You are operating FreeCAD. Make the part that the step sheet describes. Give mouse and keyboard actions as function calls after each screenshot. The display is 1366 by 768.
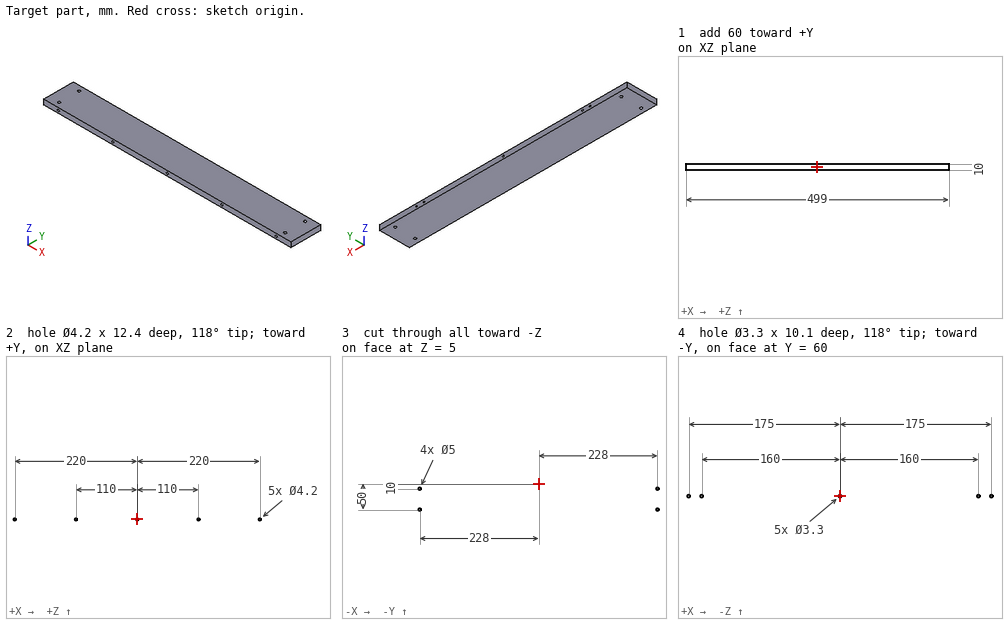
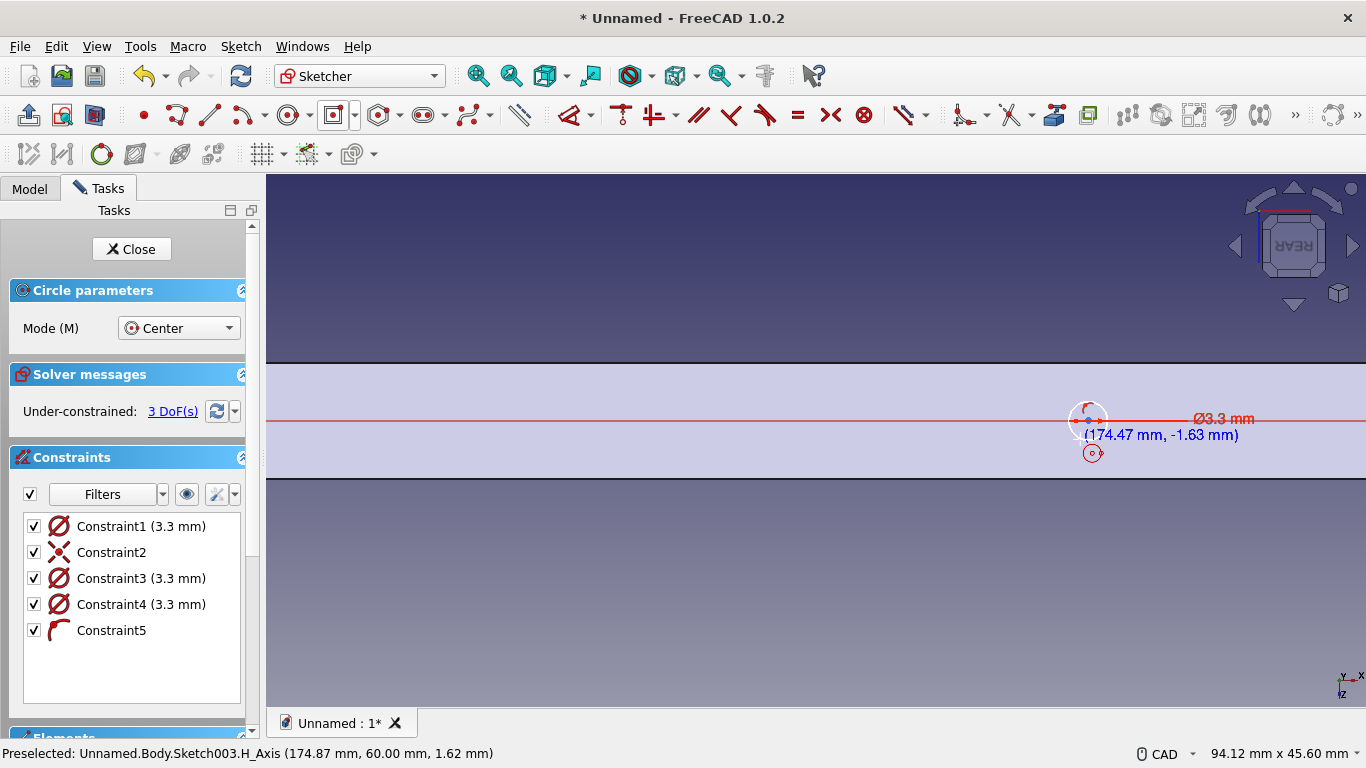
scroll(1085, 444, down, 9)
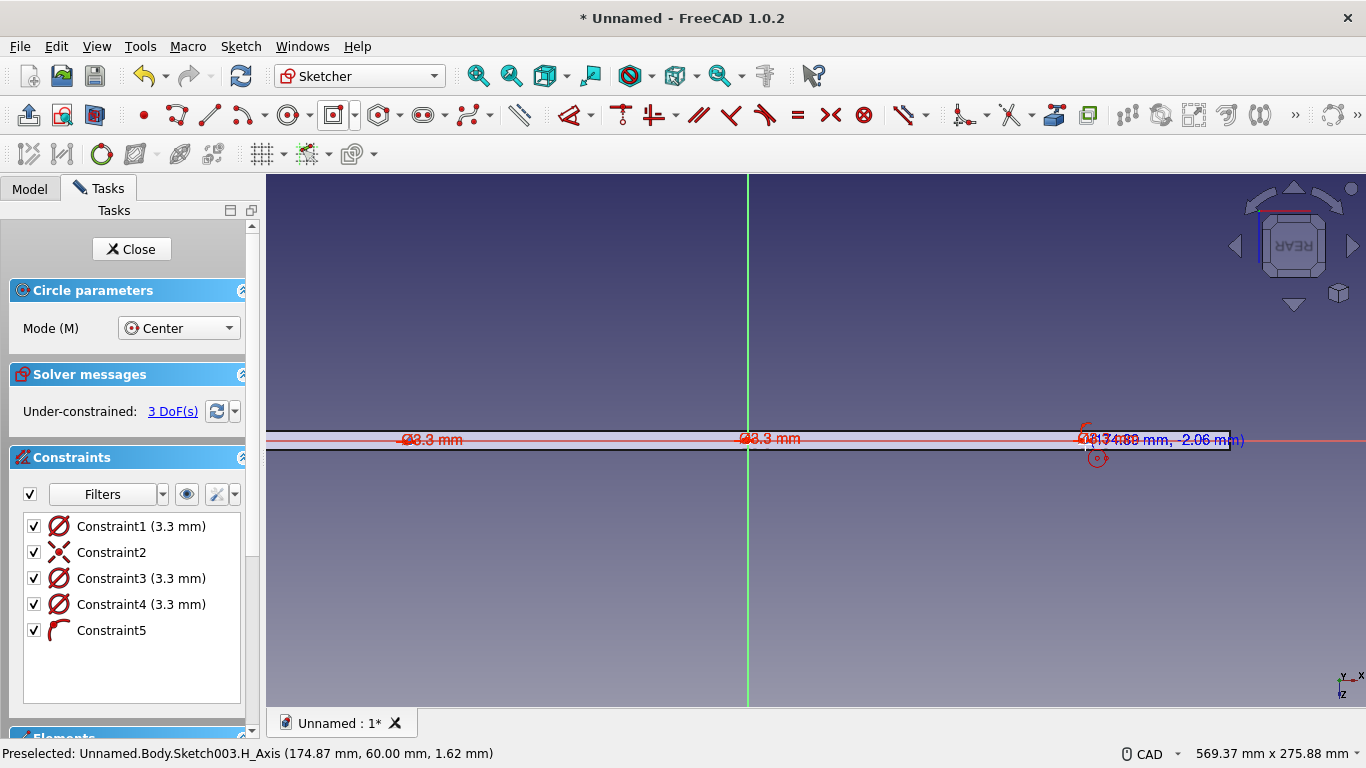
scroll(439, 441, up, 10)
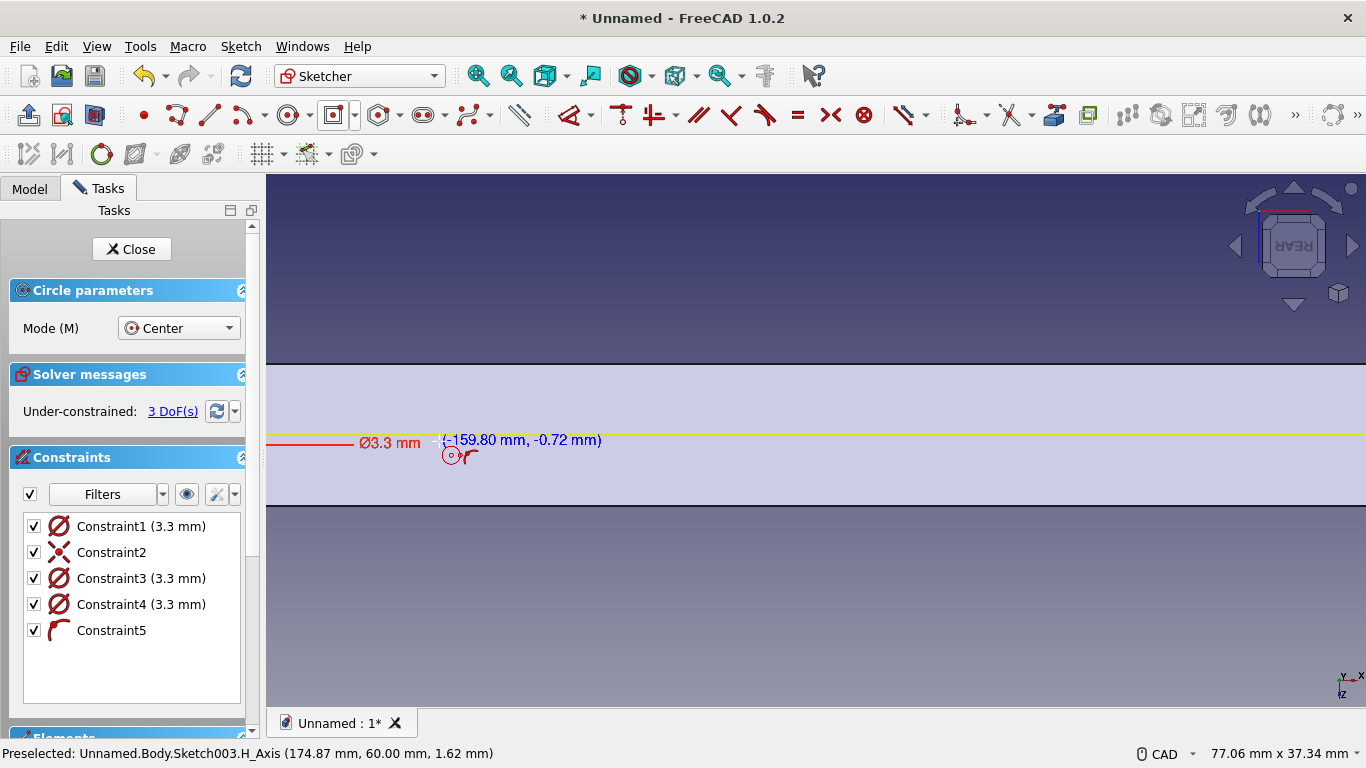
scroll(439, 441, down, 10)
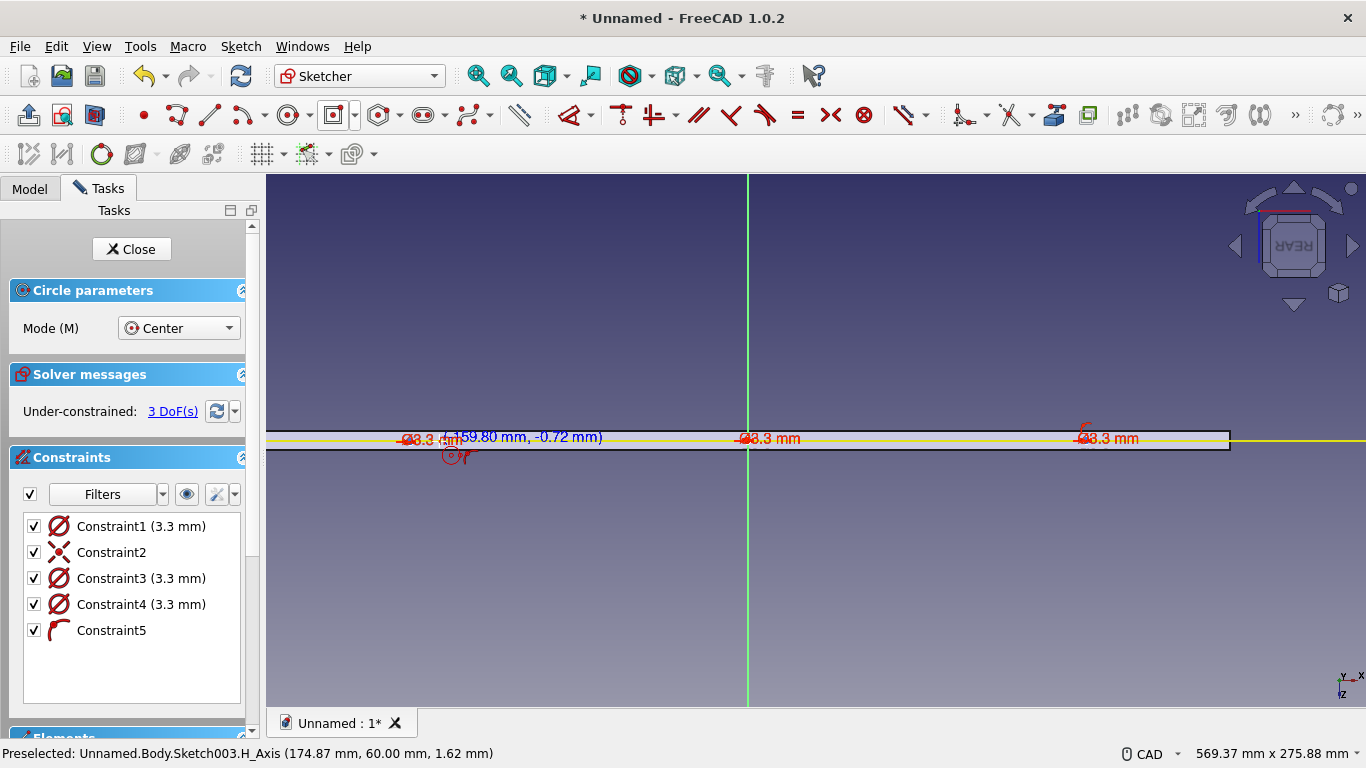
click(439, 441)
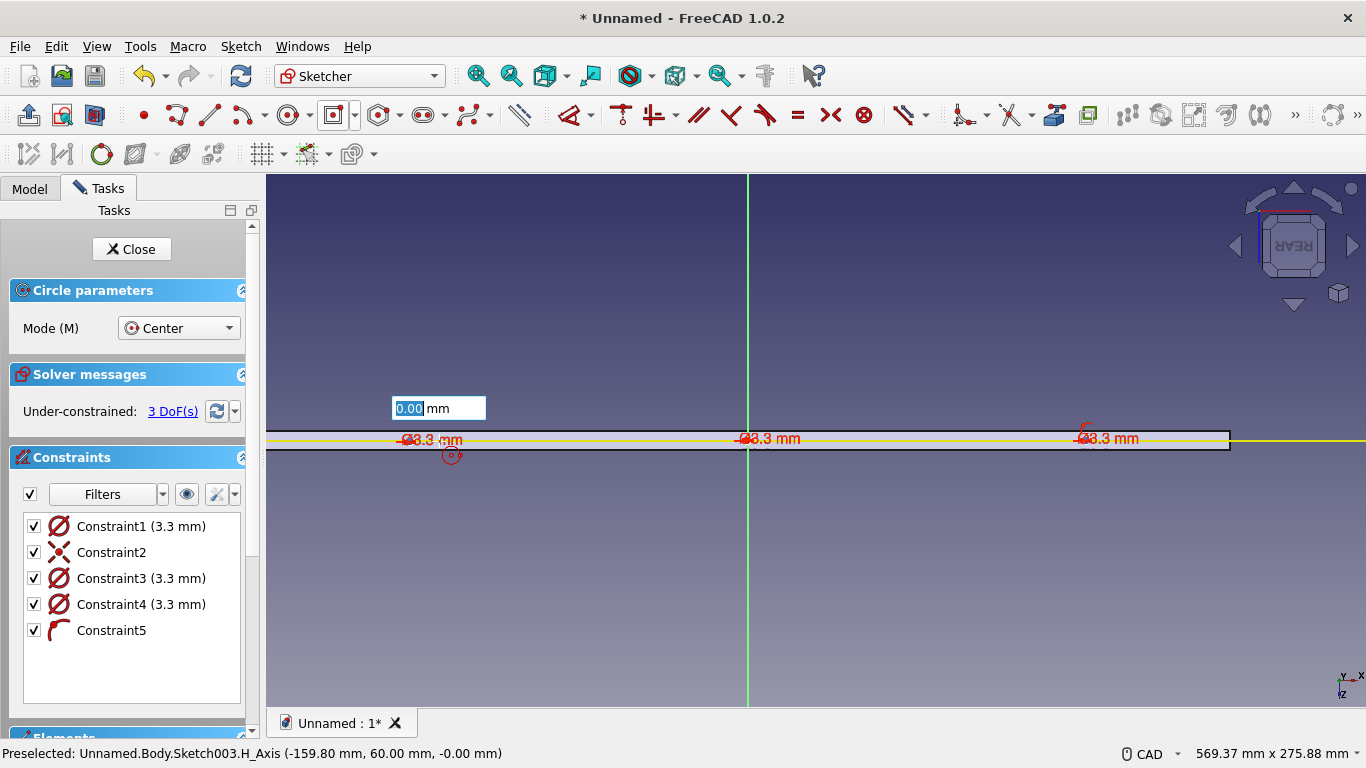
scroll(438, 444, up, 9)
move(434, 439)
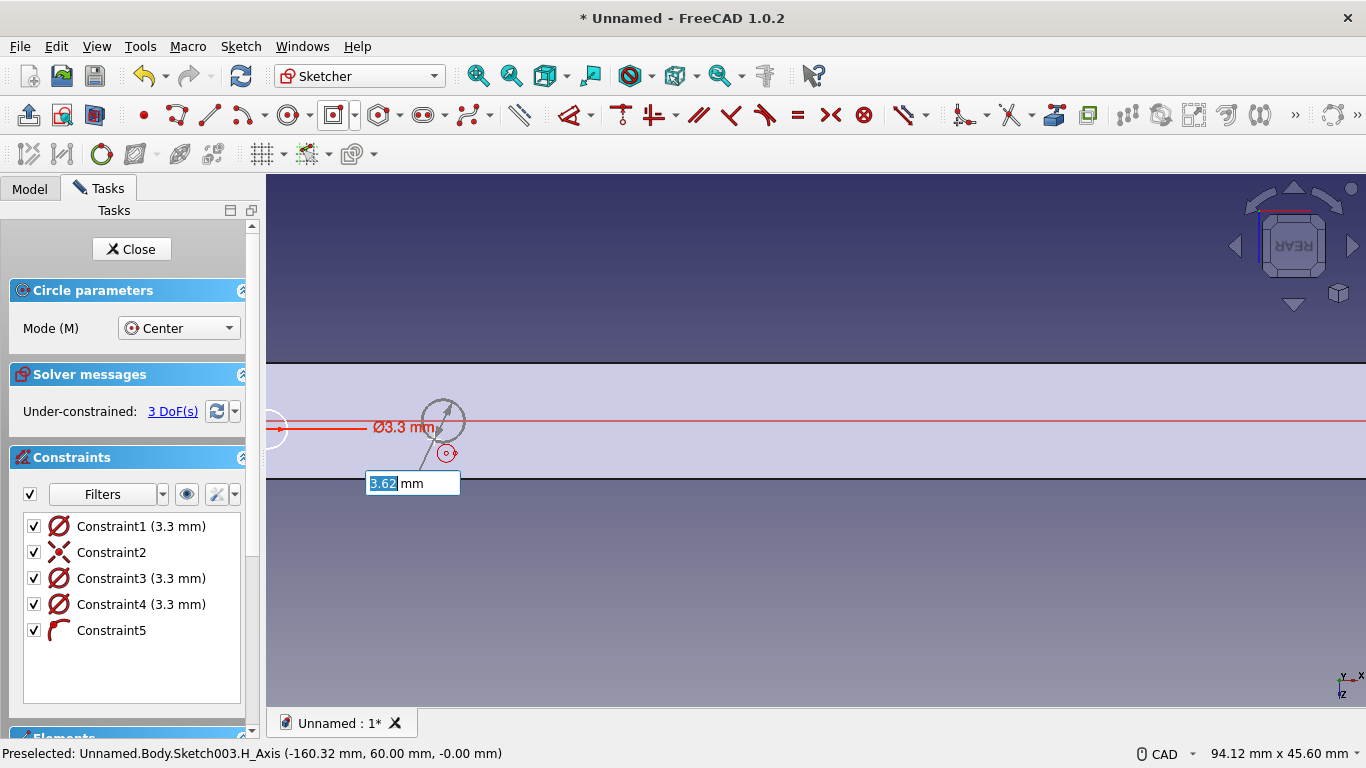
text(3.3)
key(Return)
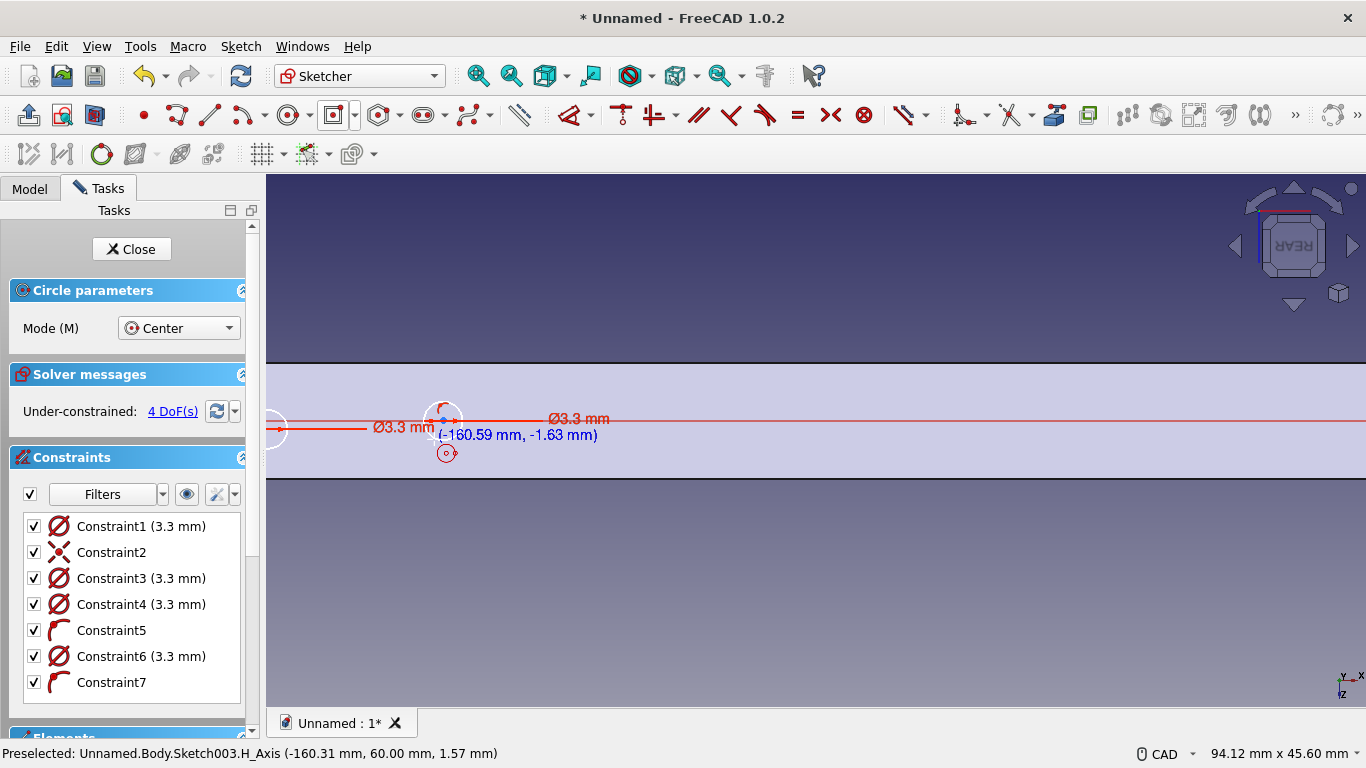
scroll(438, 444, down, 9)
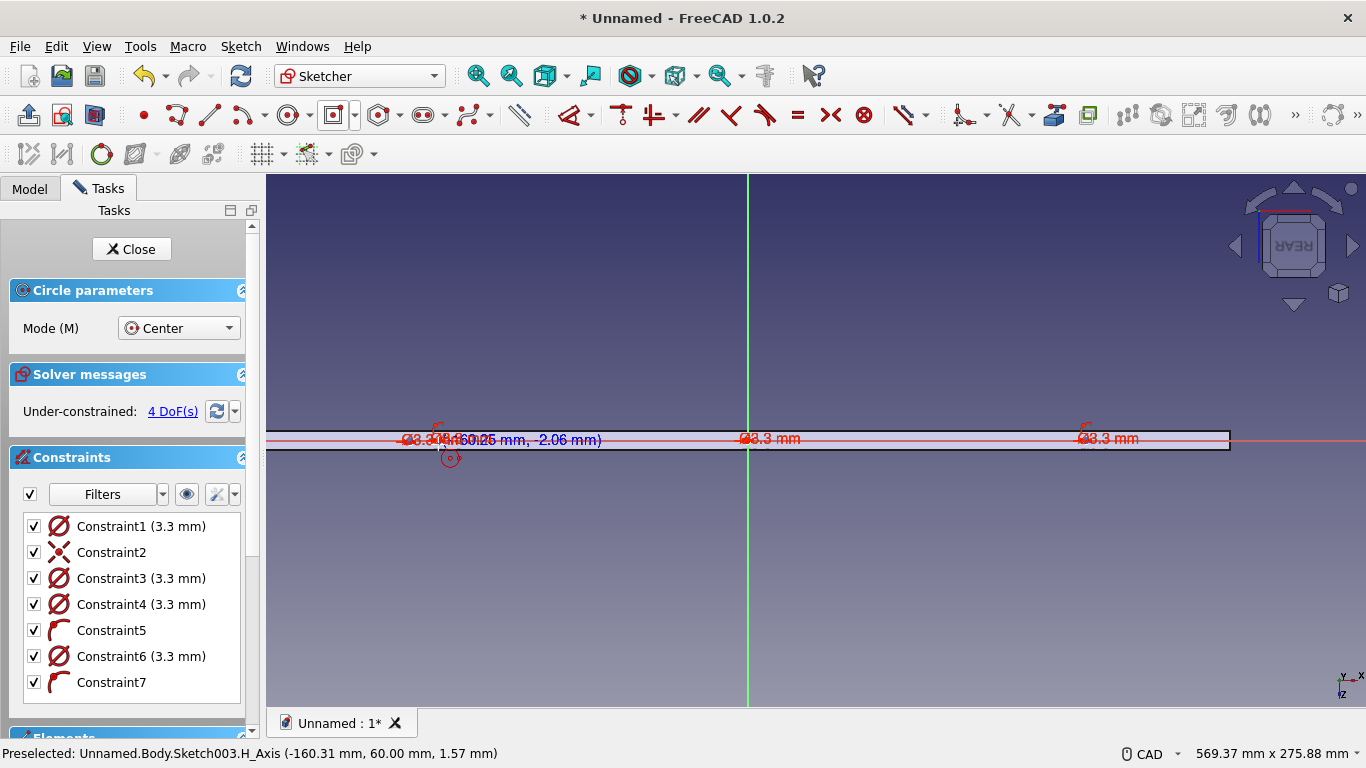
scroll(1057, 441, up, 10)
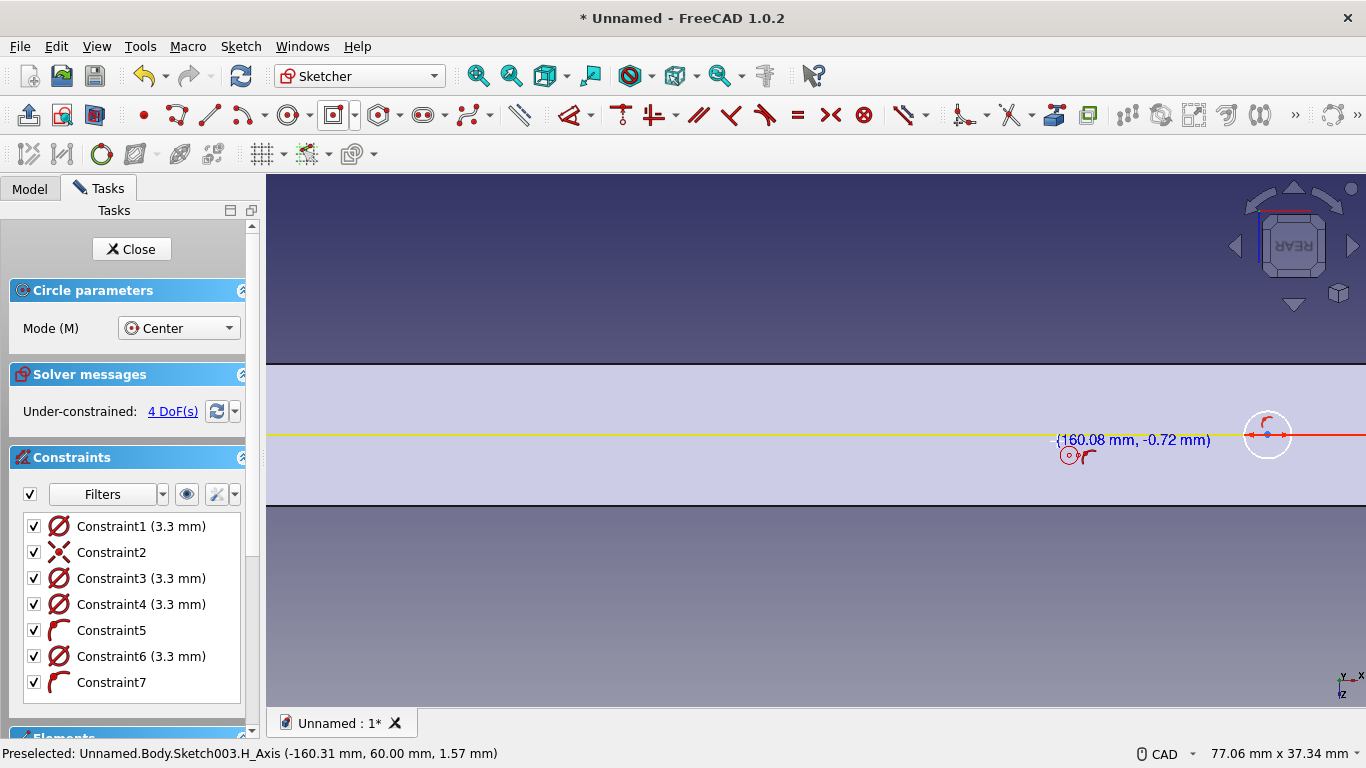
scroll(1057, 441, down, 10)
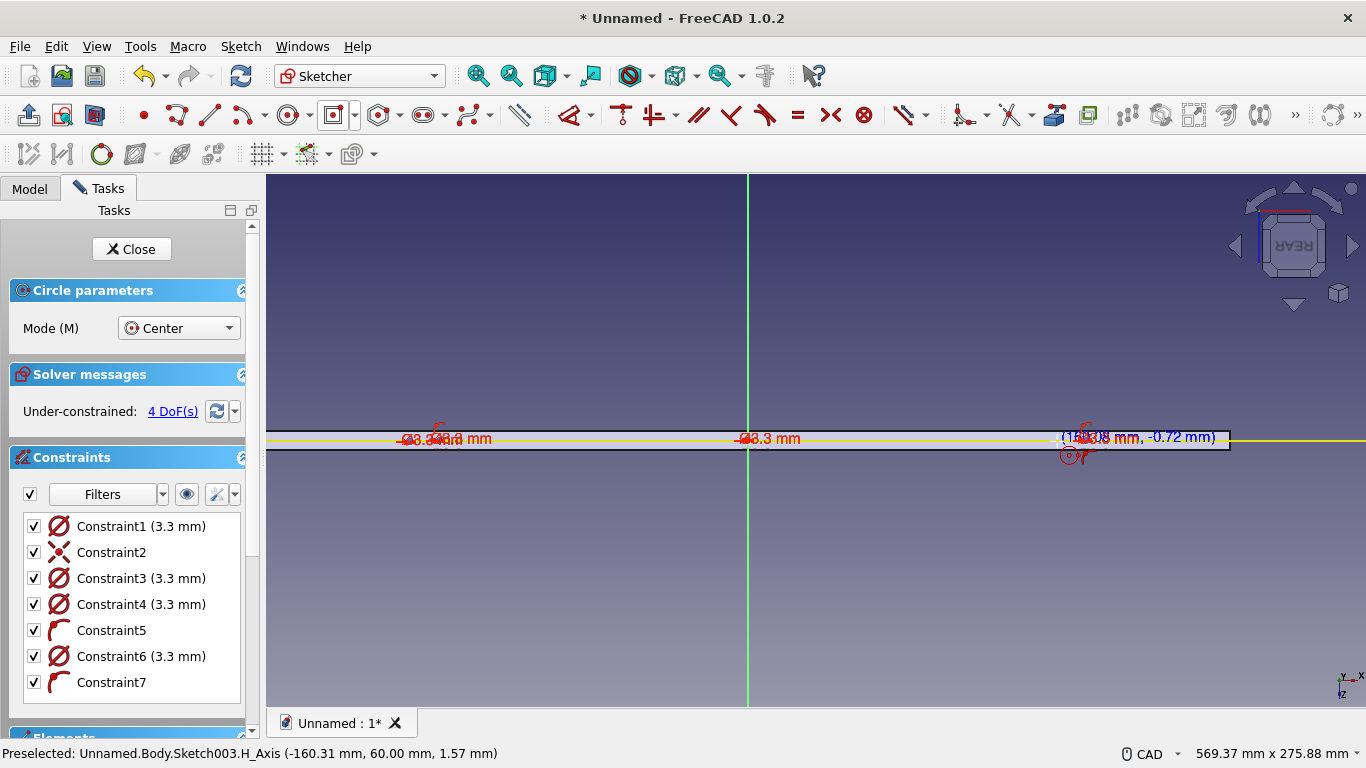
click(1057, 441)